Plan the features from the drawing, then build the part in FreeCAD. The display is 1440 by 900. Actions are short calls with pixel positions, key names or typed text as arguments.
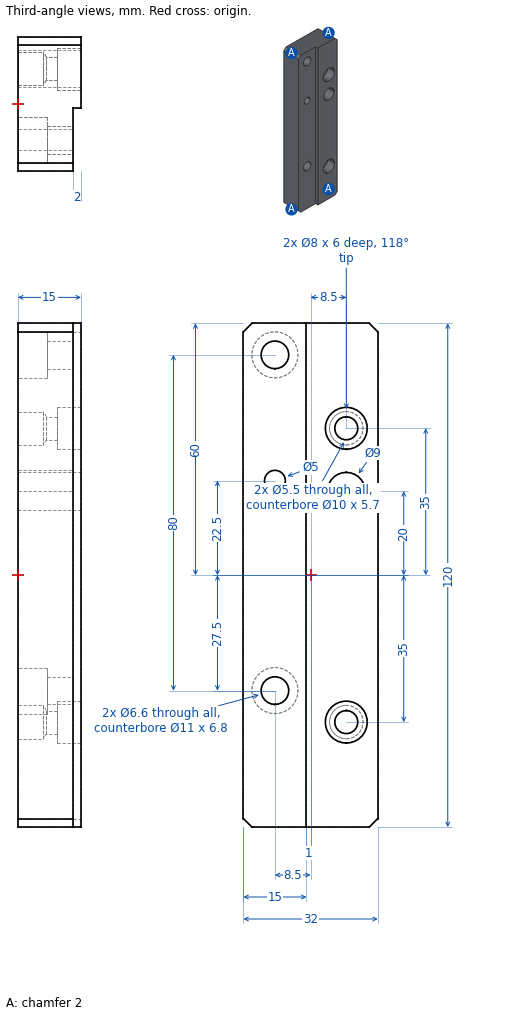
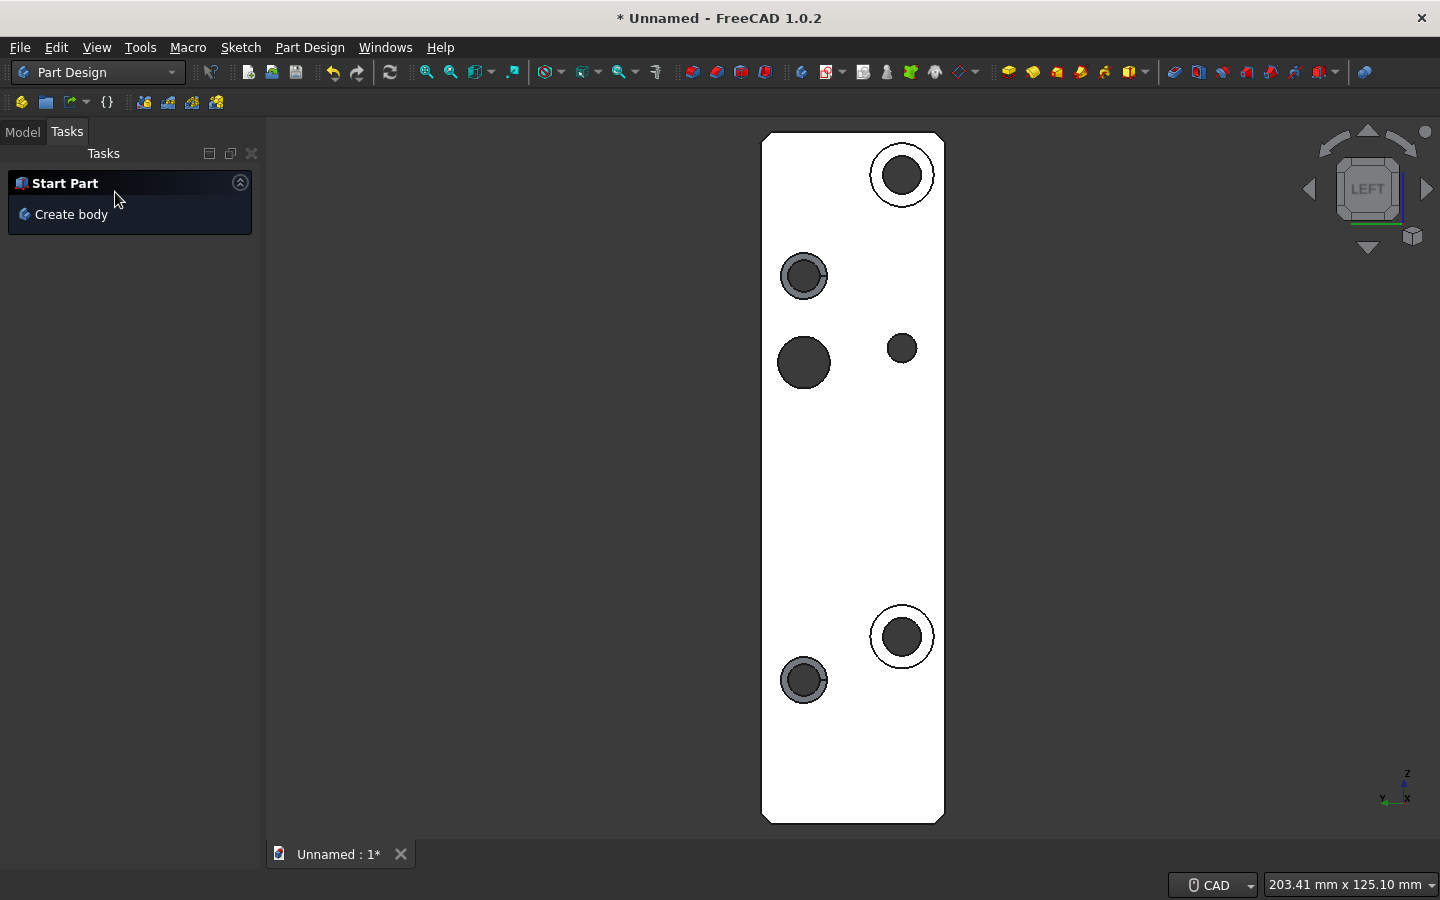
key(0)